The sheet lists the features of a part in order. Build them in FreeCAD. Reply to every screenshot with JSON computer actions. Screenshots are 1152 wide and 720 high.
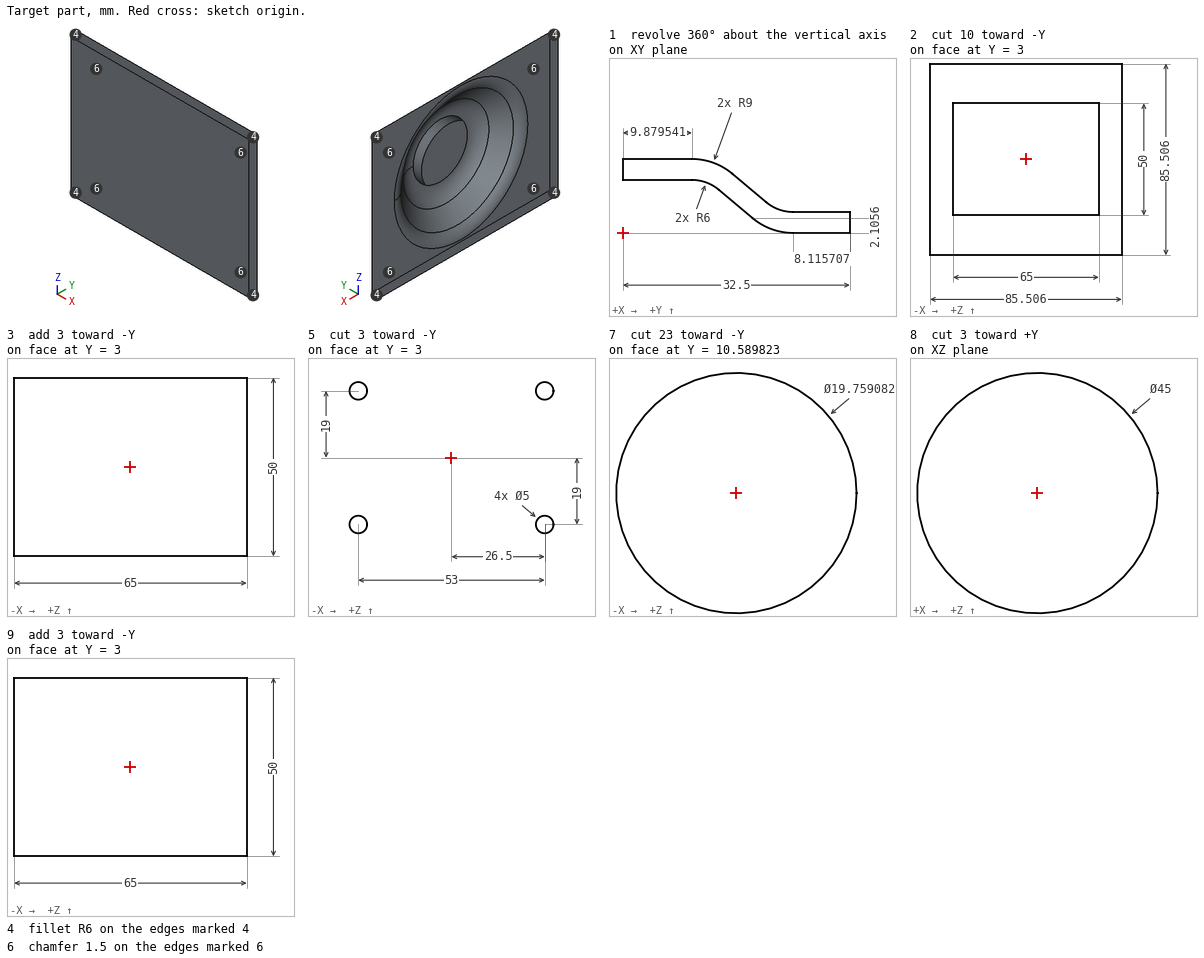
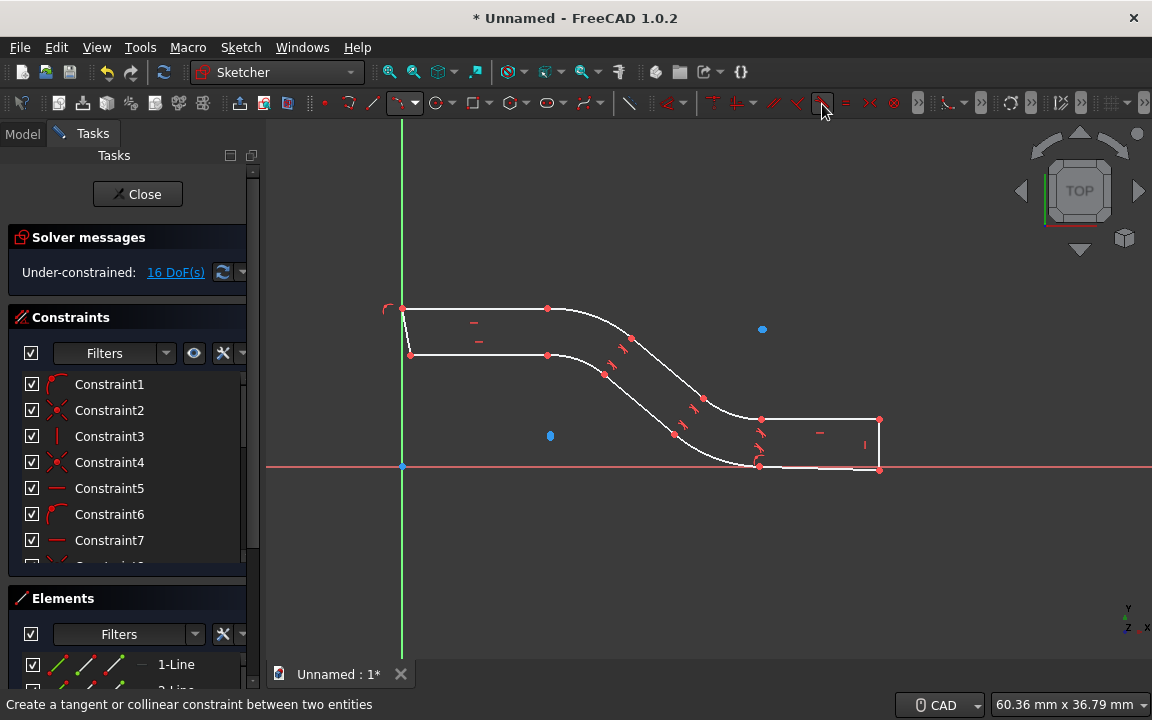
{"action": "left_click", "coordinate": [504, 309]}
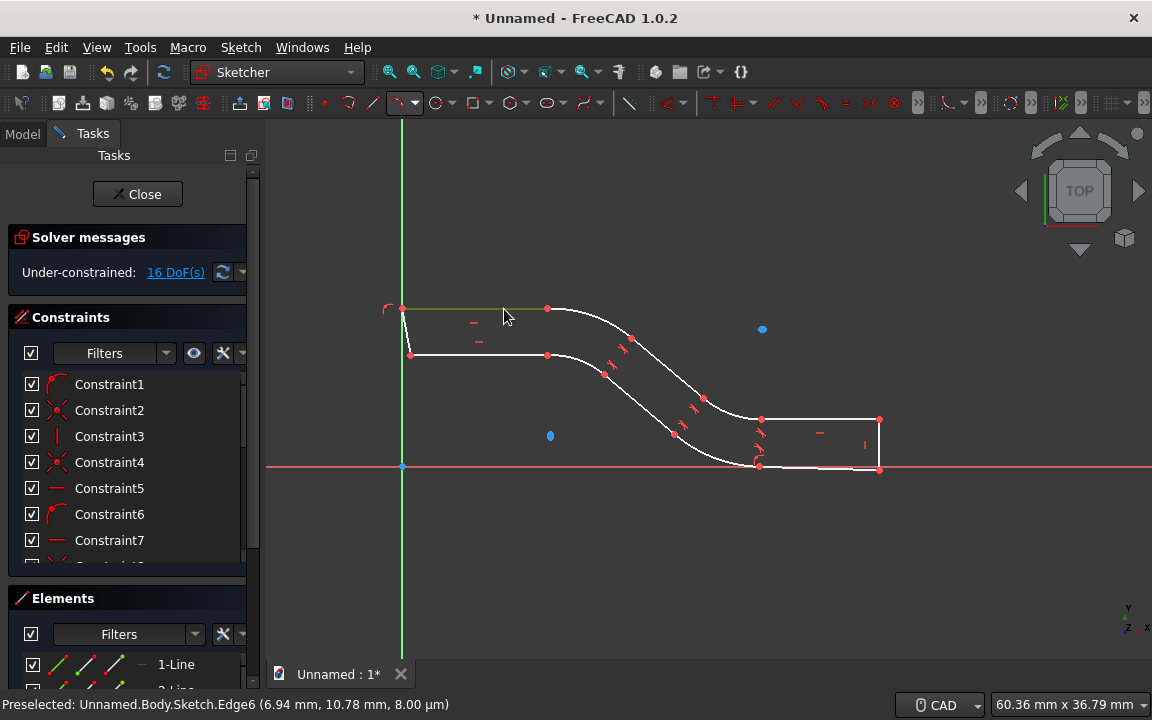
{"action": "left_click", "coordinate": [609, 323]}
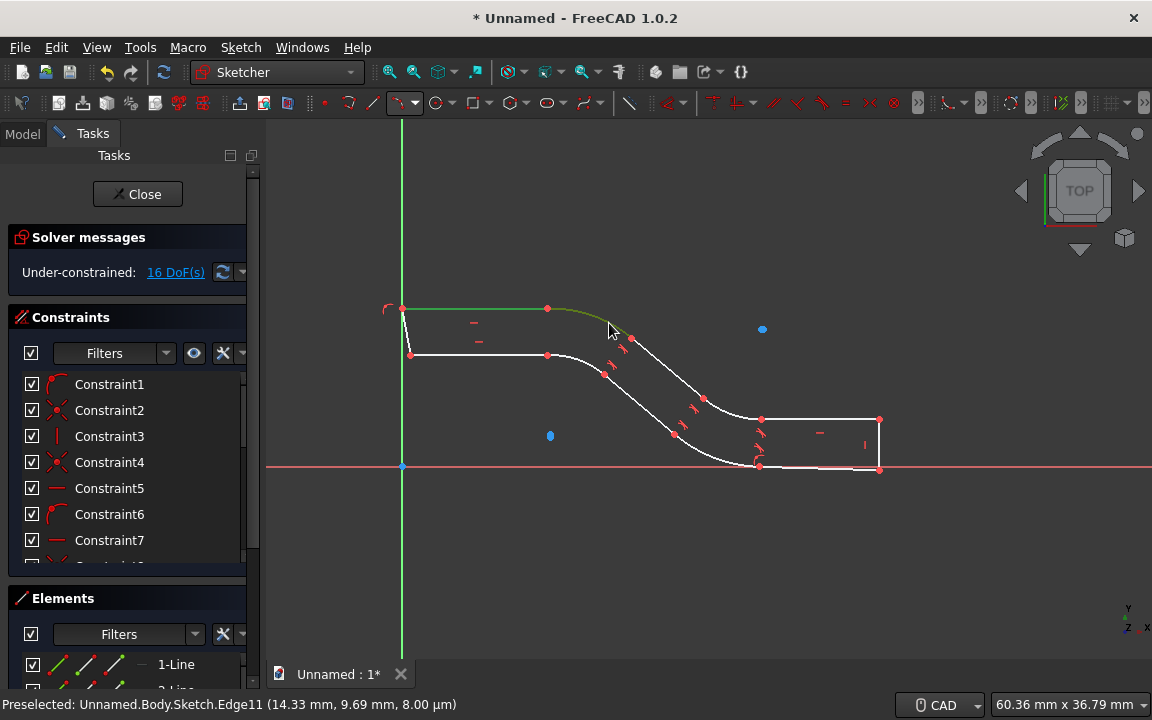
{"action": "left_click", "coordinate": [822, 104]}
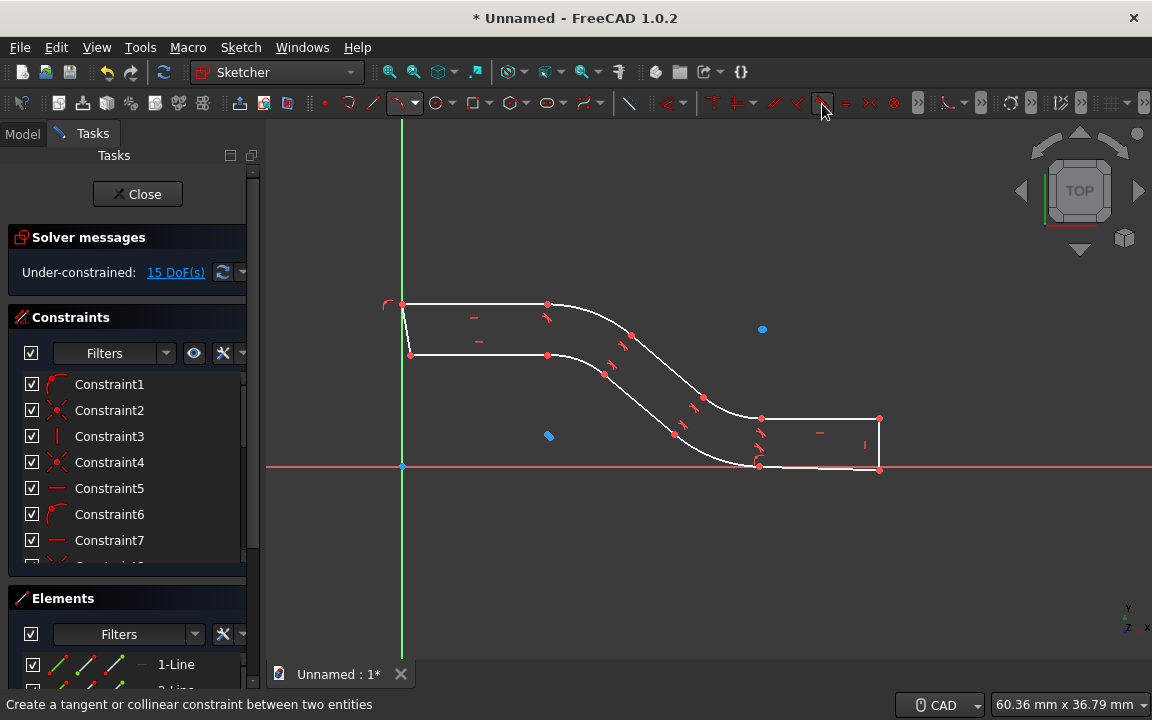
{"action": "left_click", "coordinate": [452, 355]}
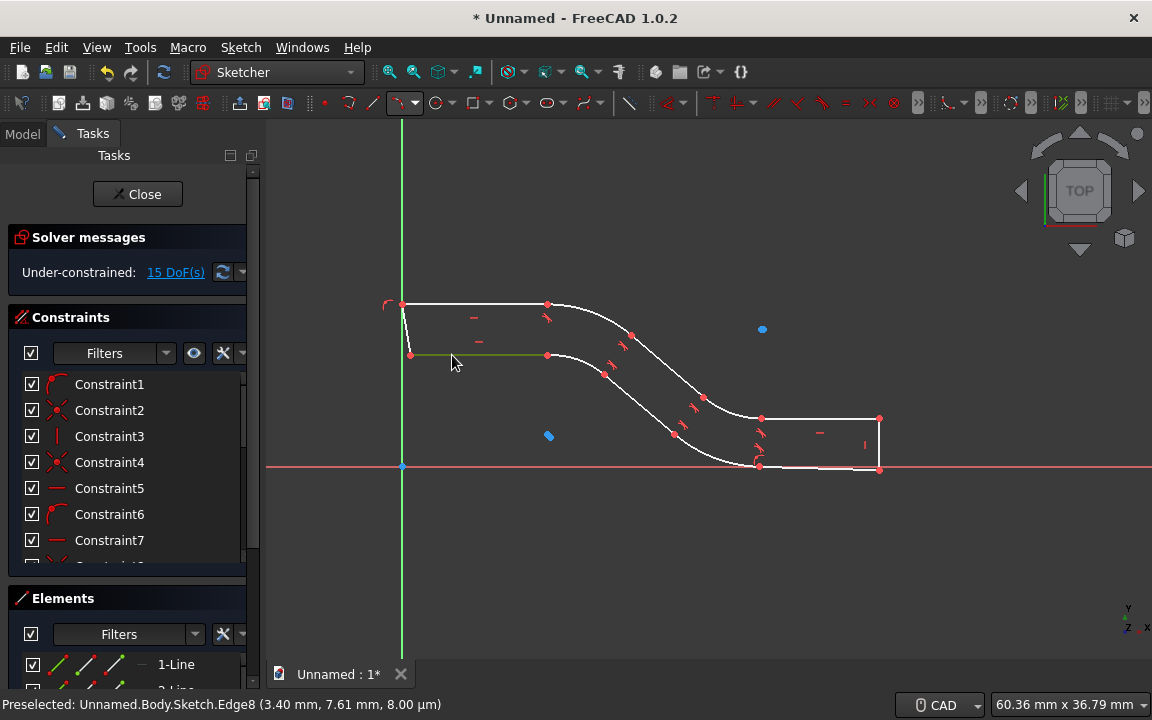
{"action": "left_click", "coordinate": [589, 364]}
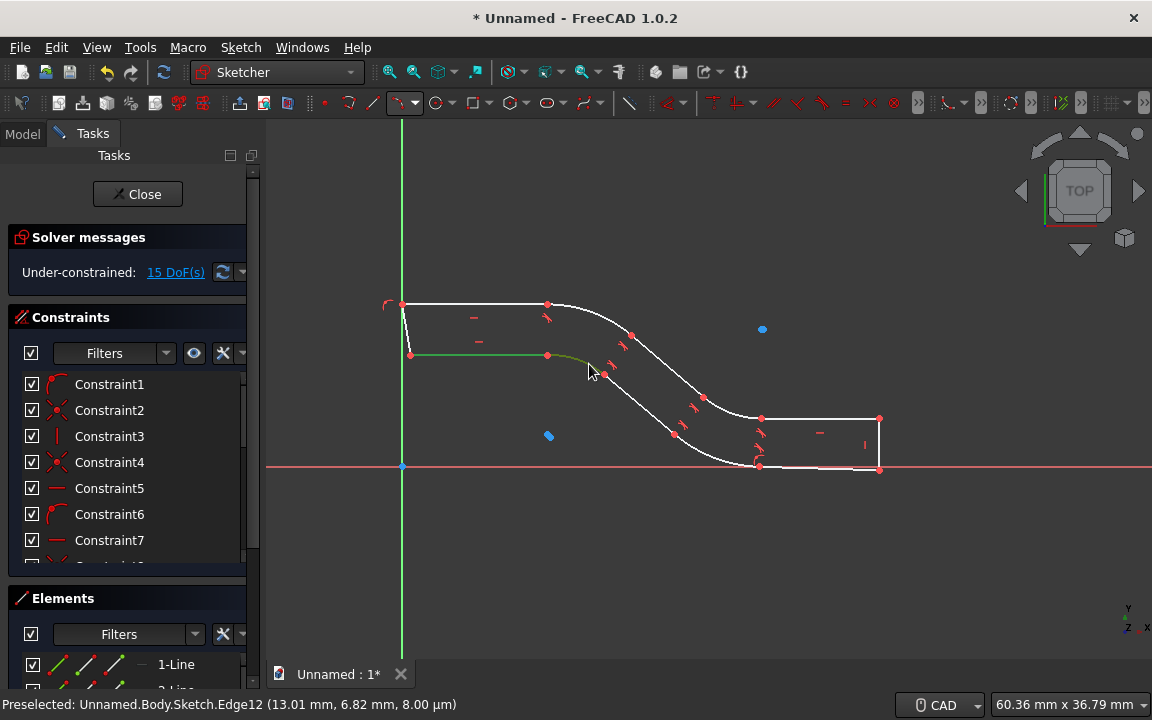
{"action": "left_click", "coordinate": [822, 104]}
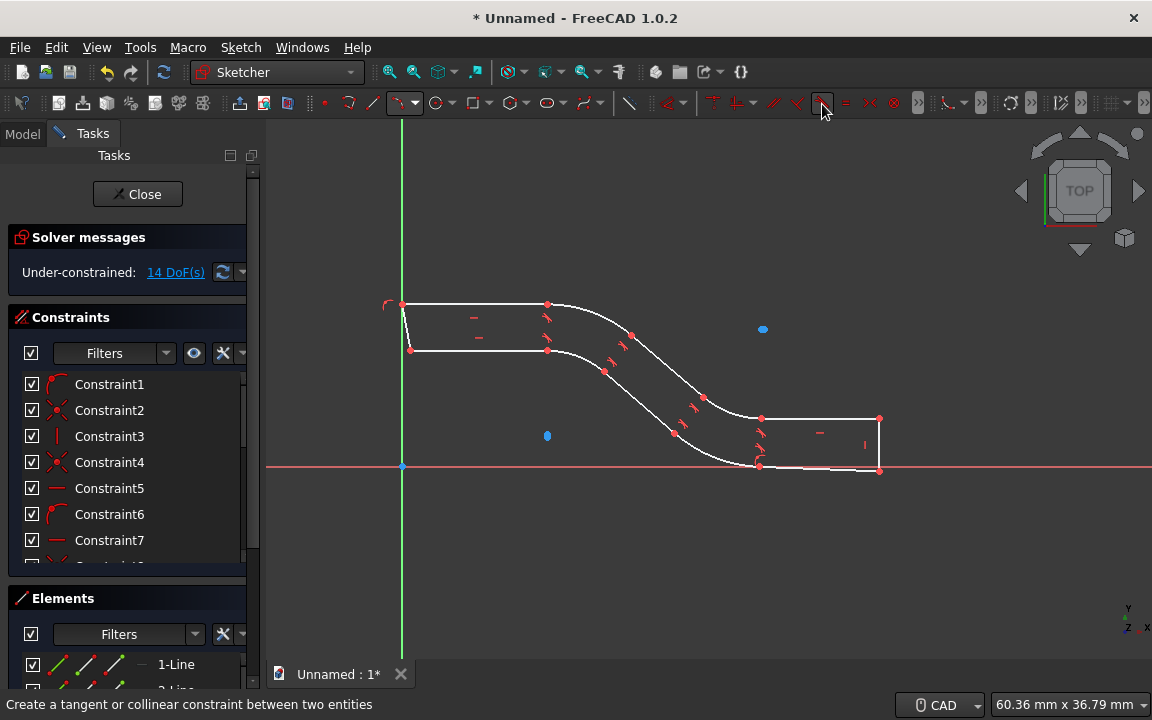
{"action": "left_click", "coordinate": [795, 468]}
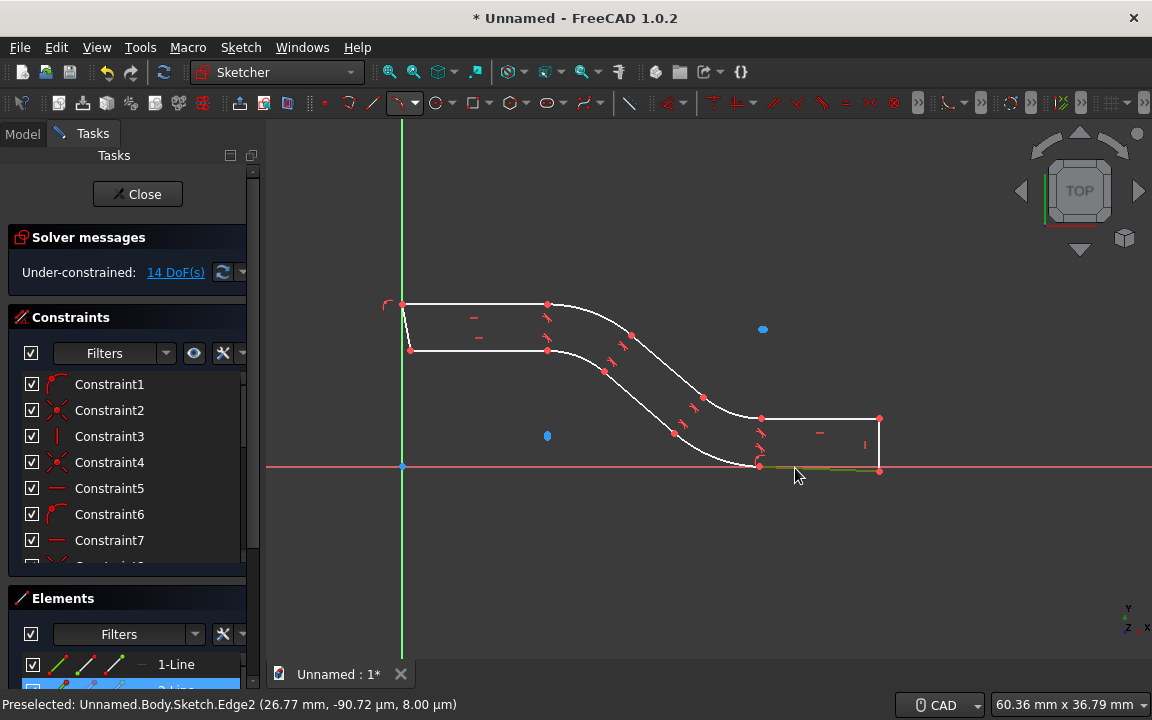
{"action": "key", "text": "h"}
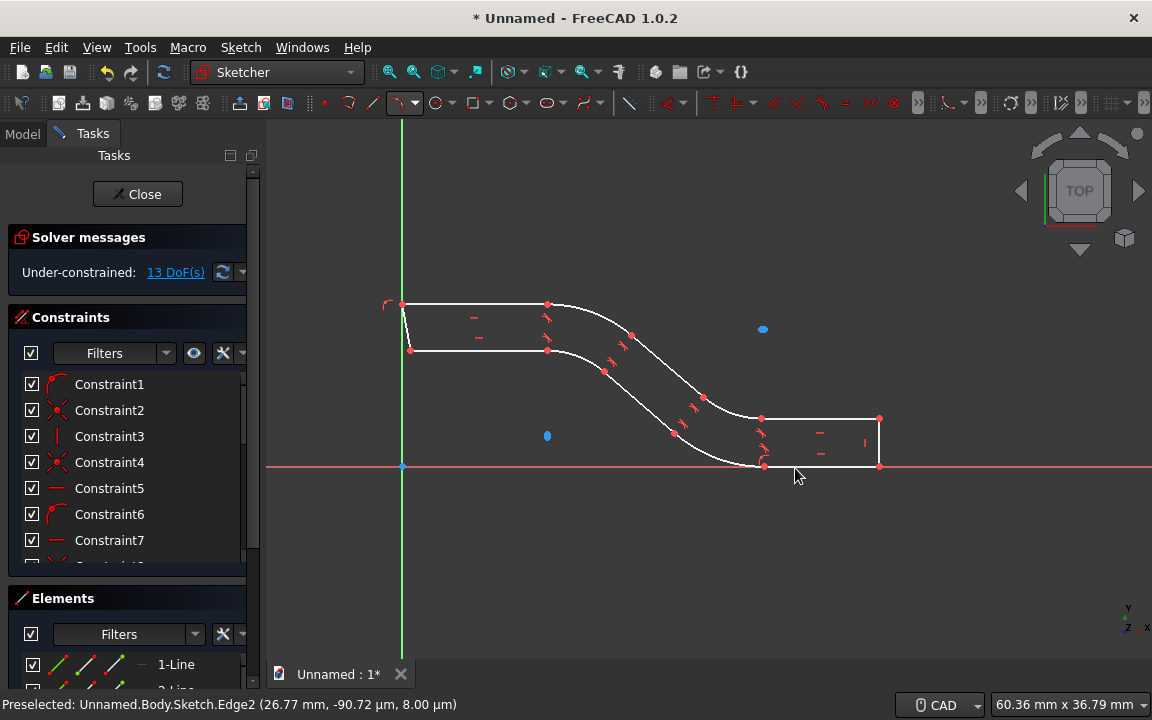
{"action": "left_click", "coordinate": [405, 318]}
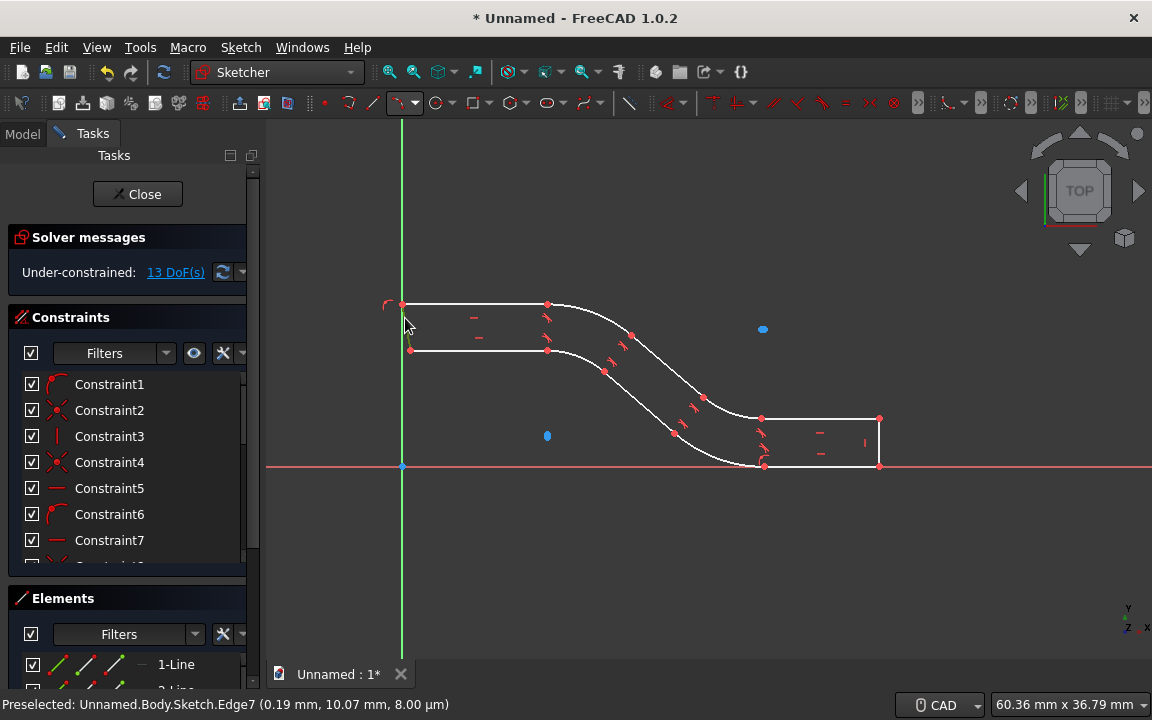
{"action": "left_click", "coordinate": [756, 104]}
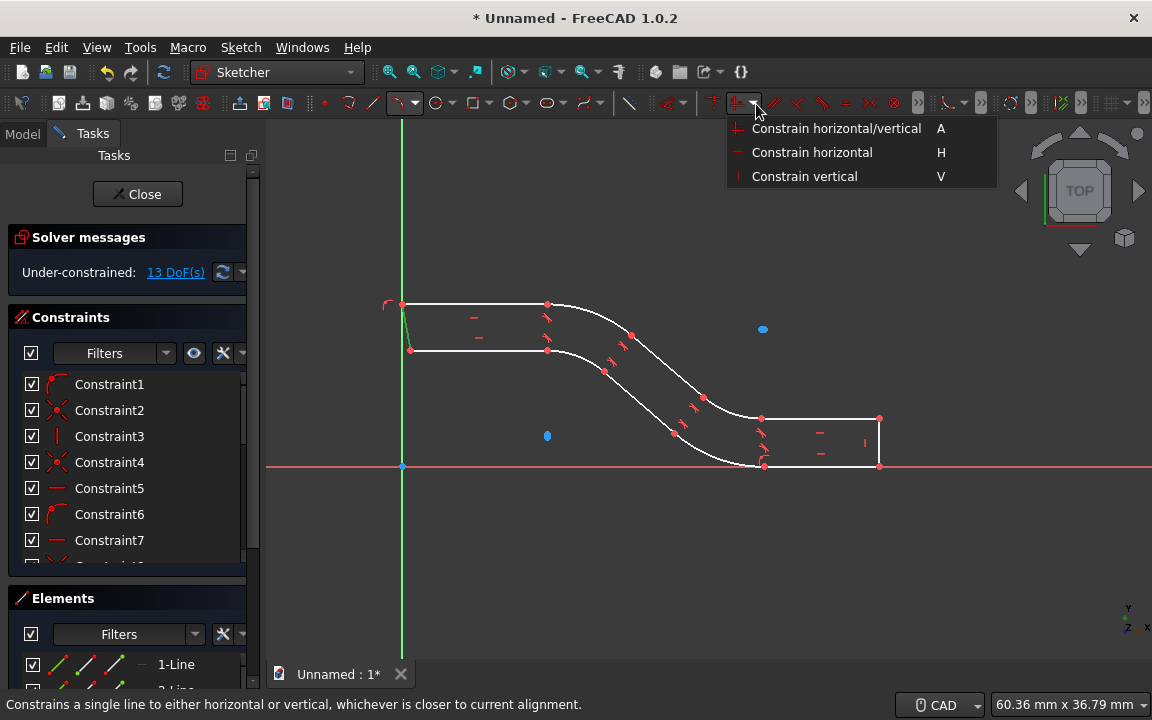
{"action": "left_click", "coordinate": [862, 176]}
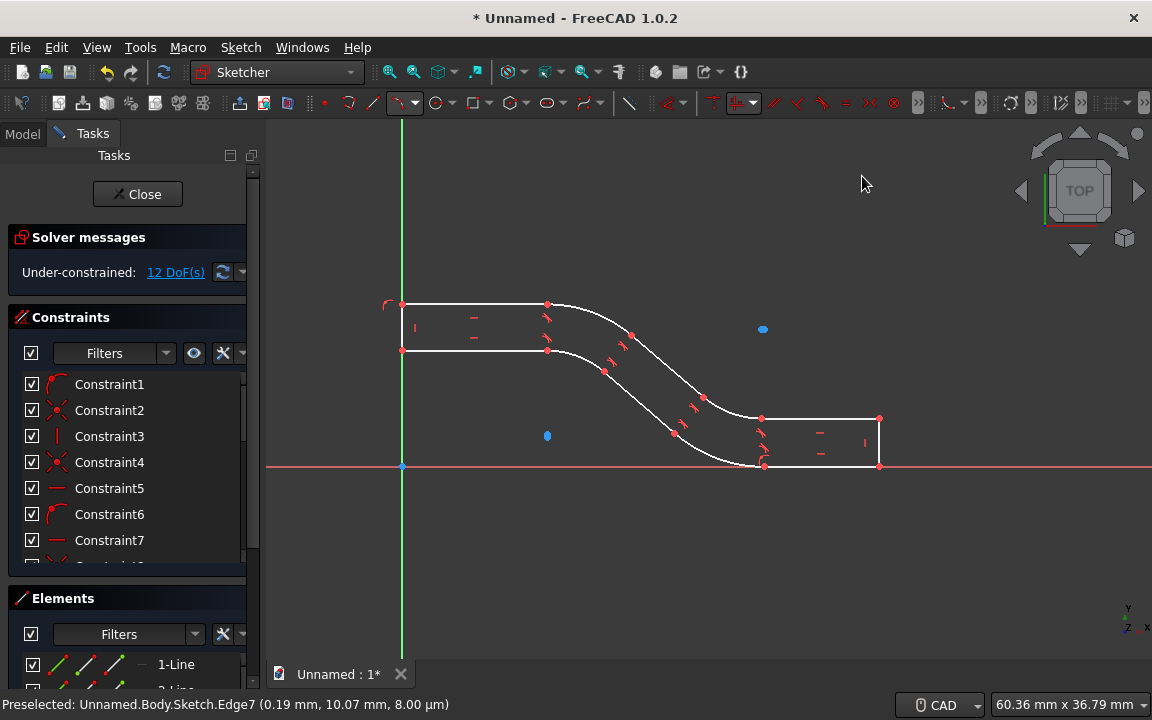
{"action": "left_click", "coordinate": [699, 450]}